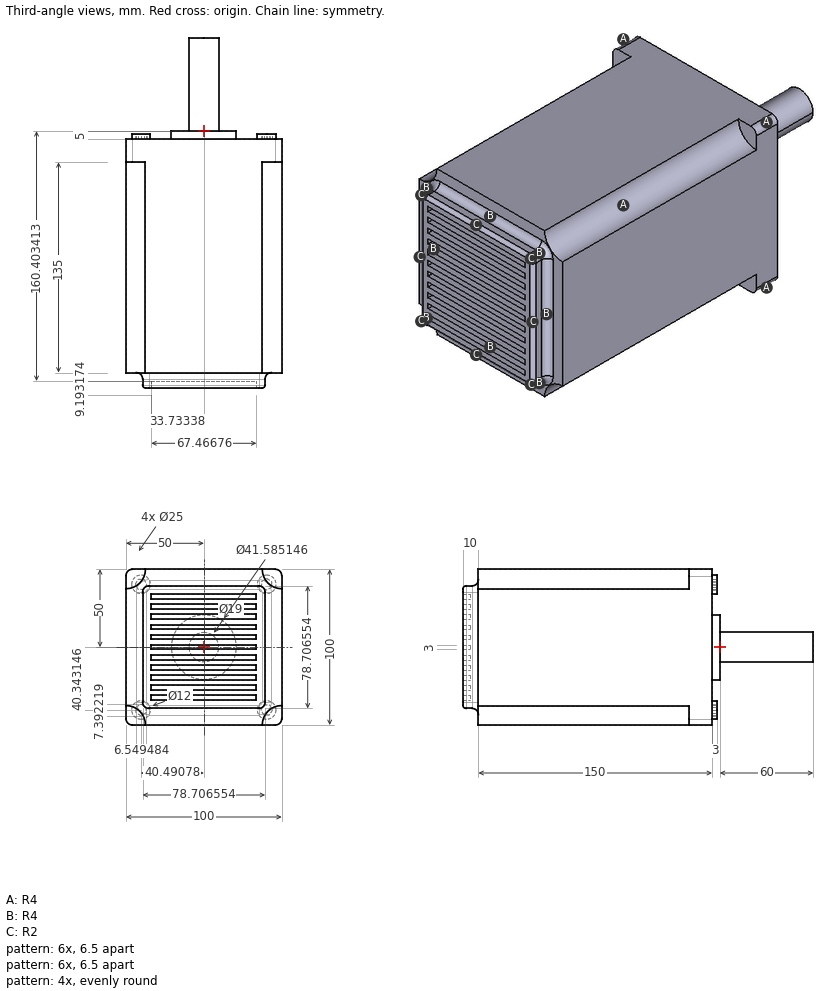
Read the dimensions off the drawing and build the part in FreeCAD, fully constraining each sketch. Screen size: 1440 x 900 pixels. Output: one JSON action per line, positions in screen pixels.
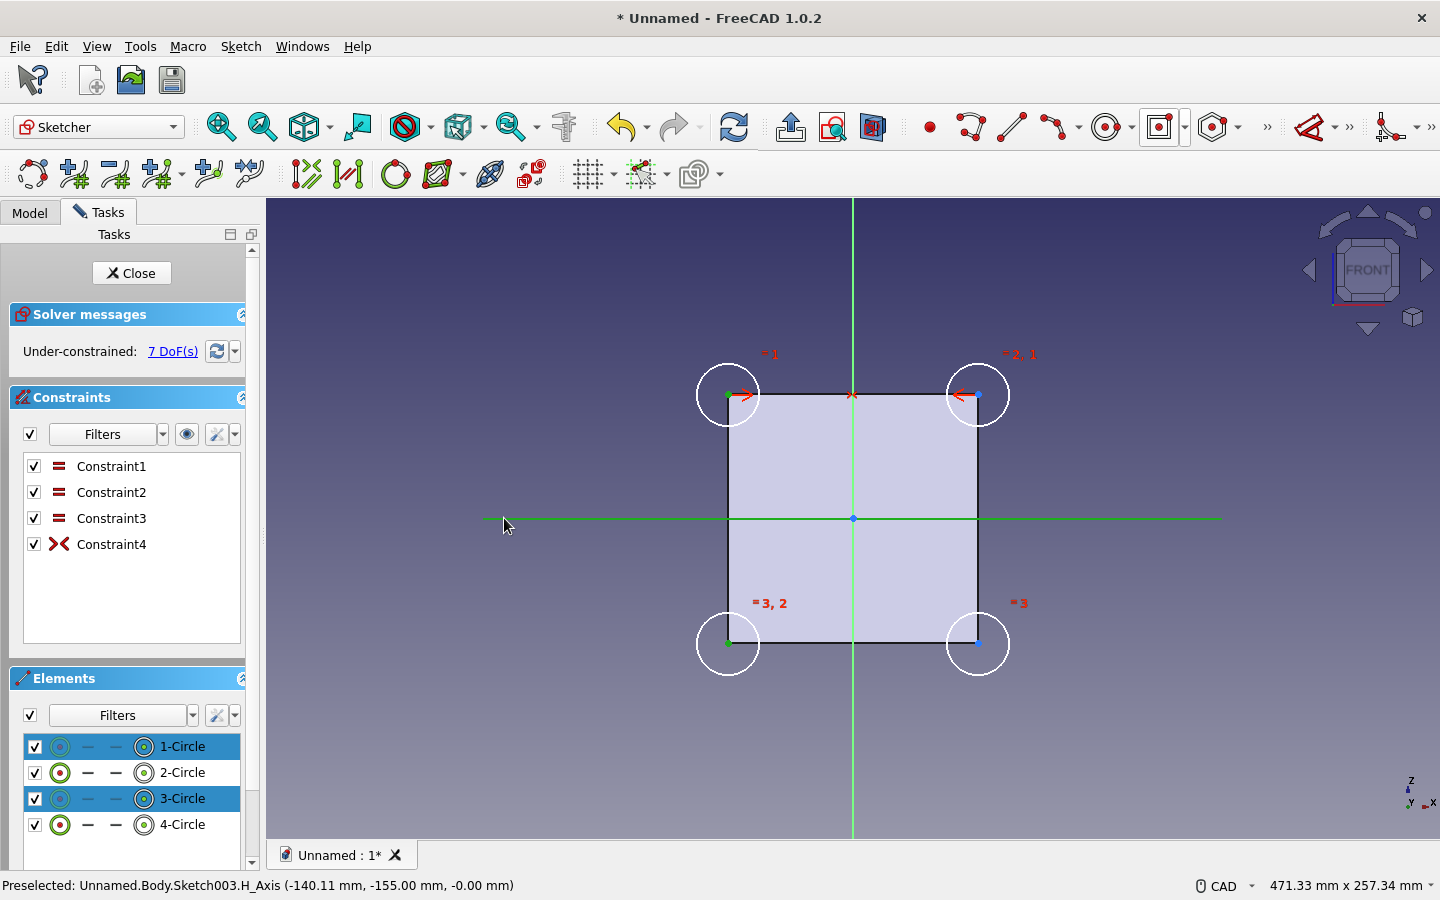
{"action": "key", "text": "s"}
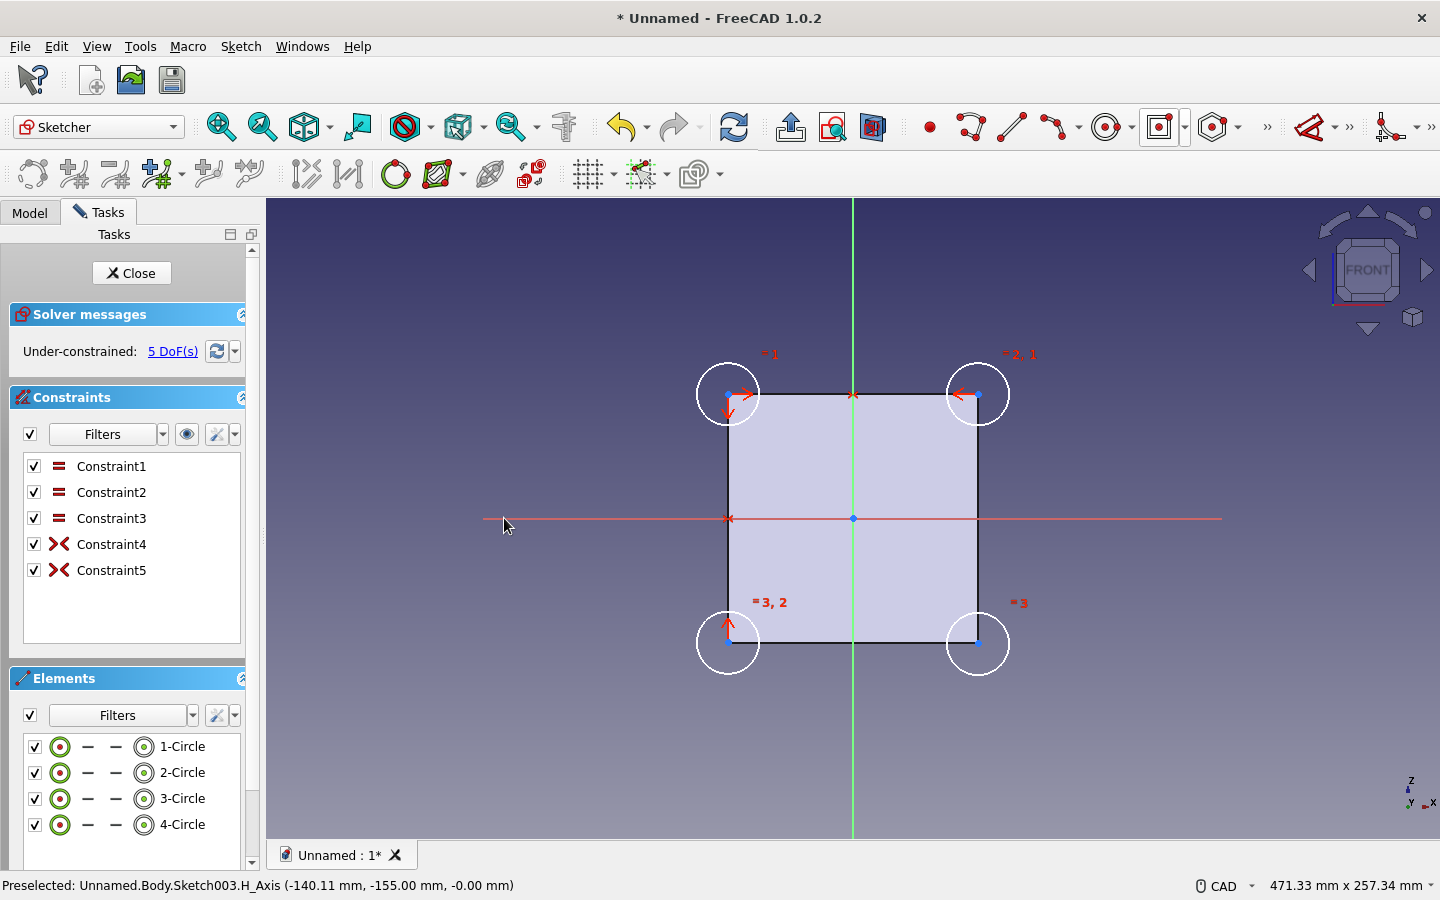
{"action": "left_click", "coordinate": [978, 394]}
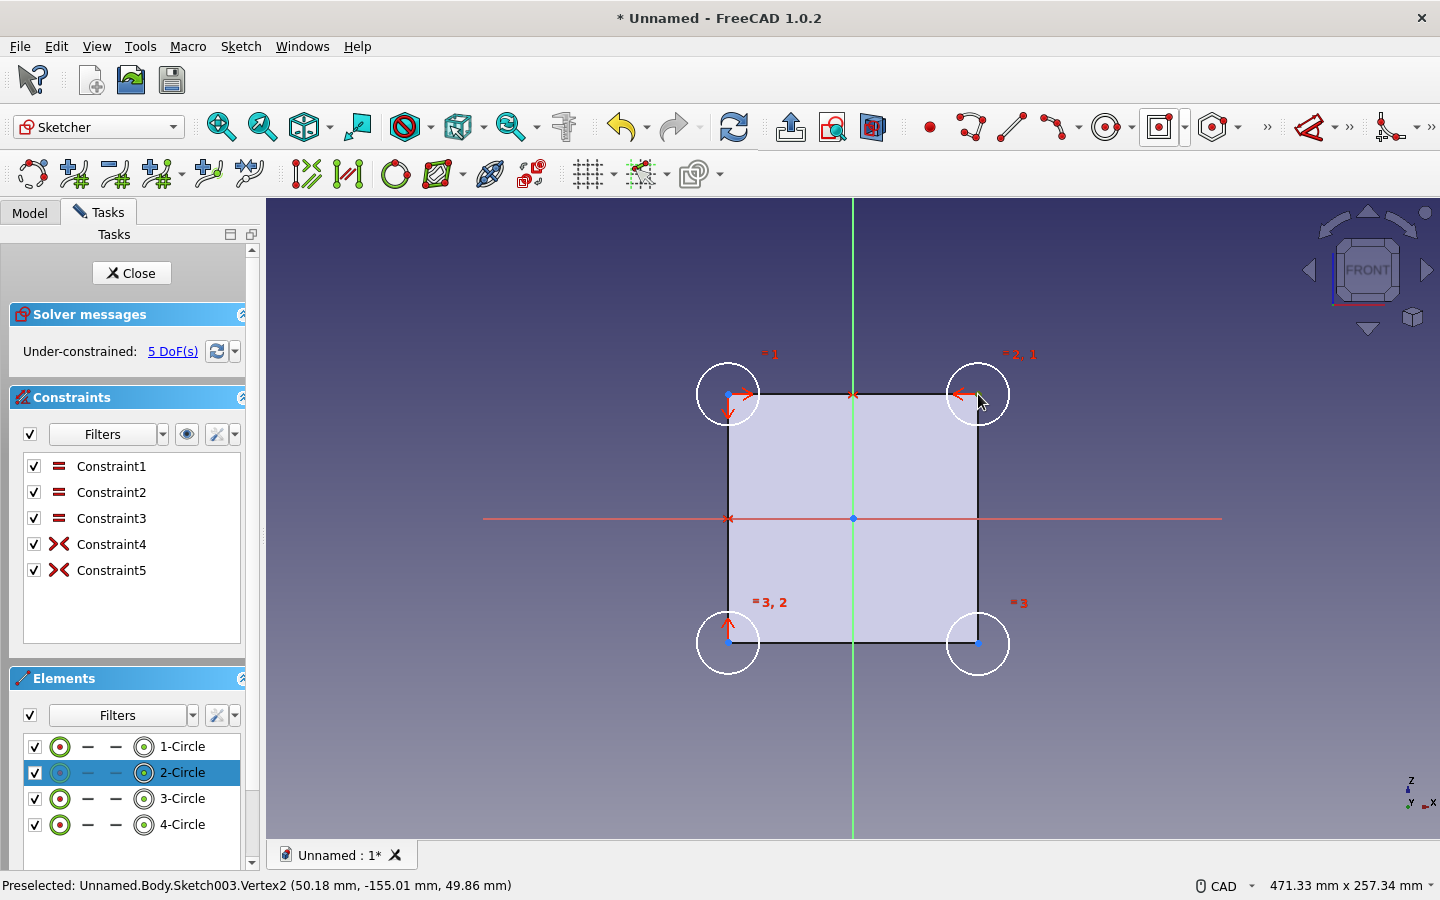
{"action": "left_click", "coordinate": [978, 644]}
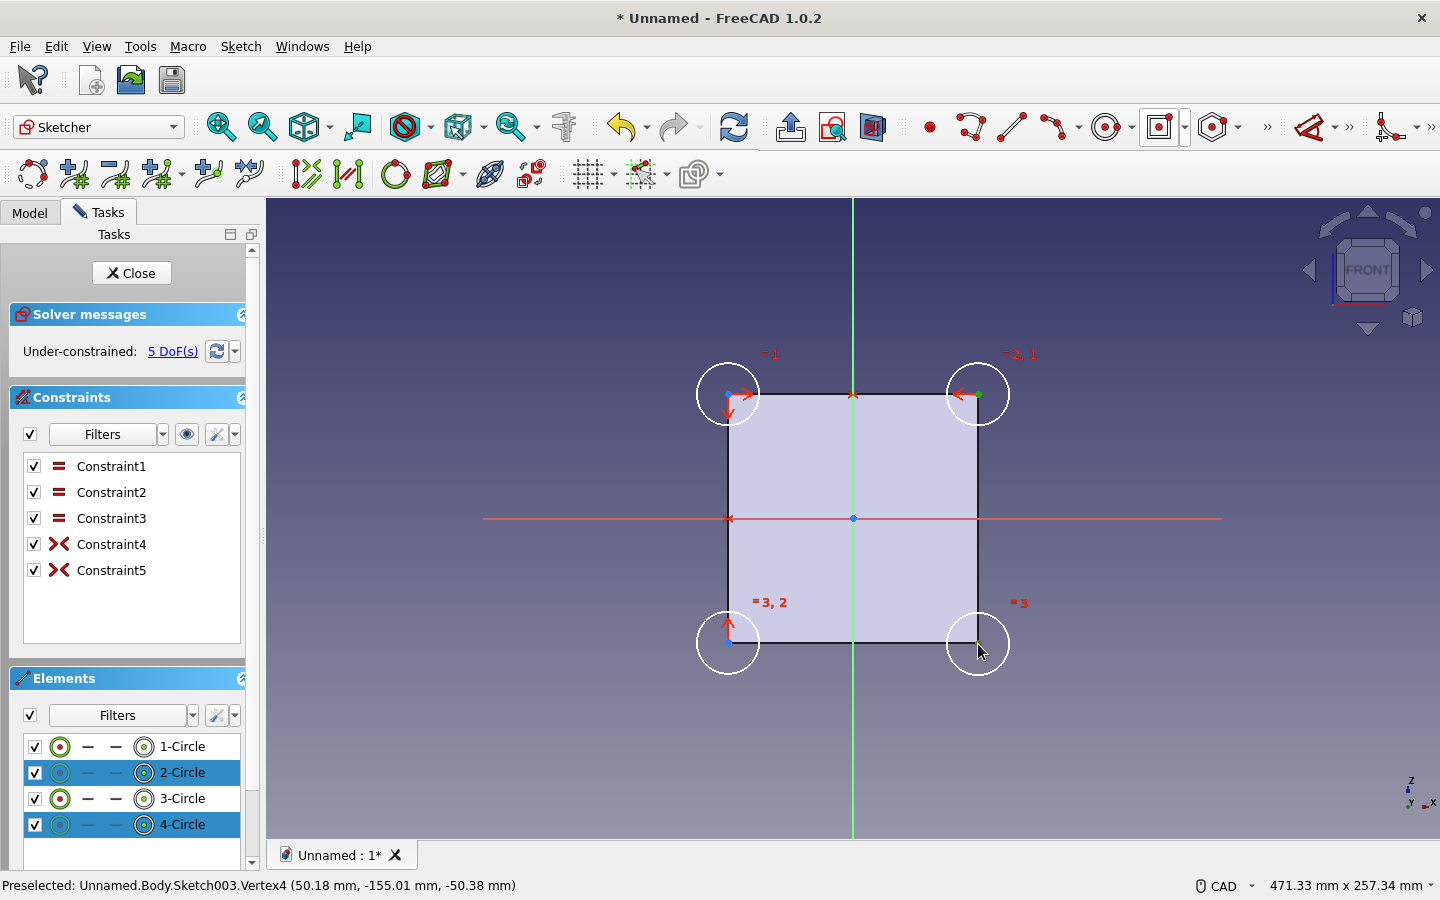
{"action": "left_click", "coordinate": [504, 518]}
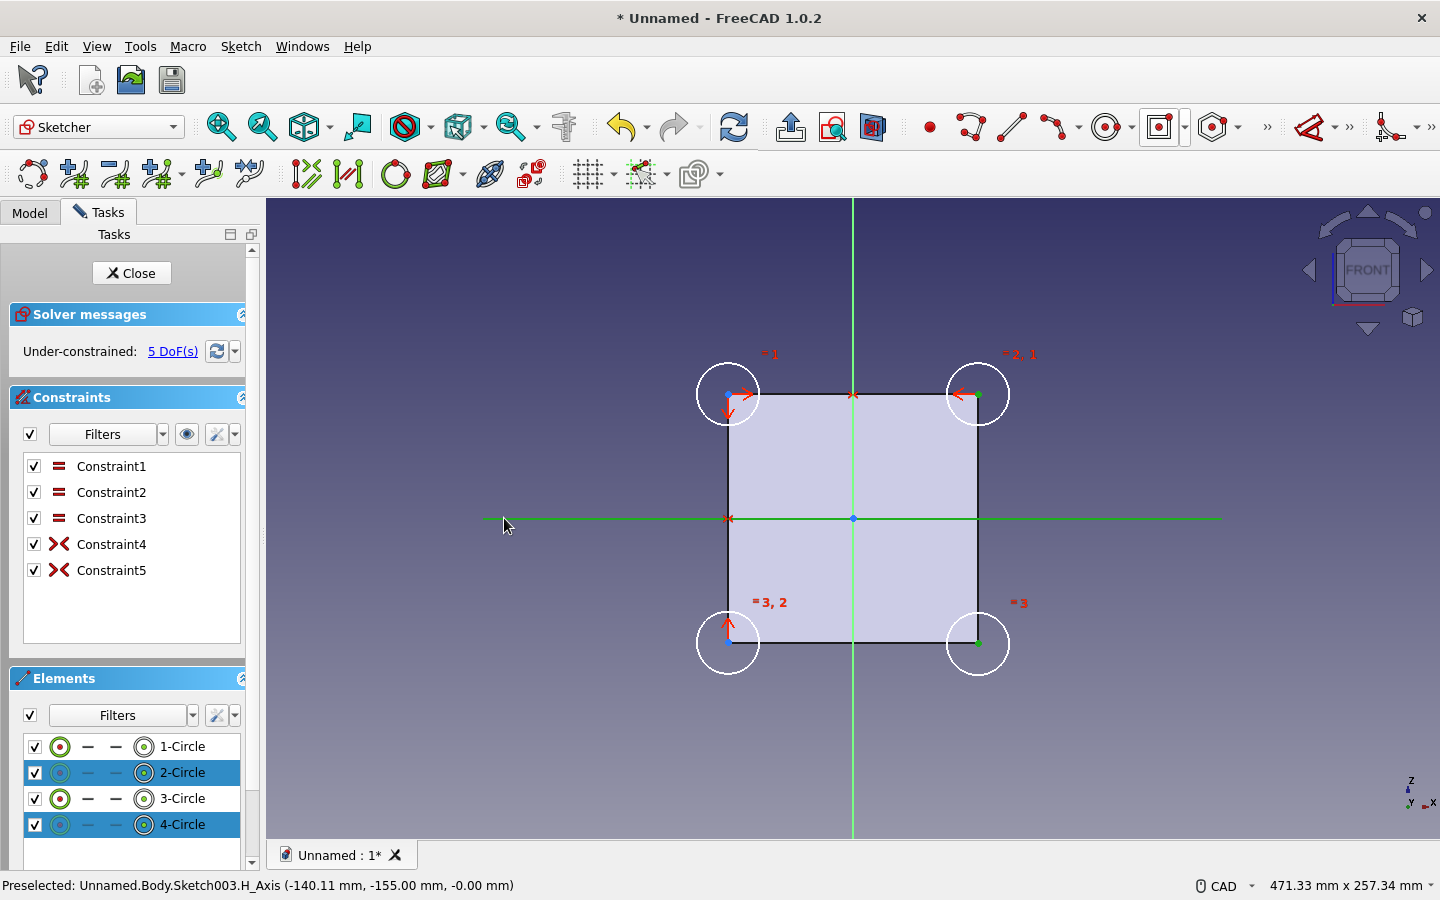
{"action": "key", "text": "s"}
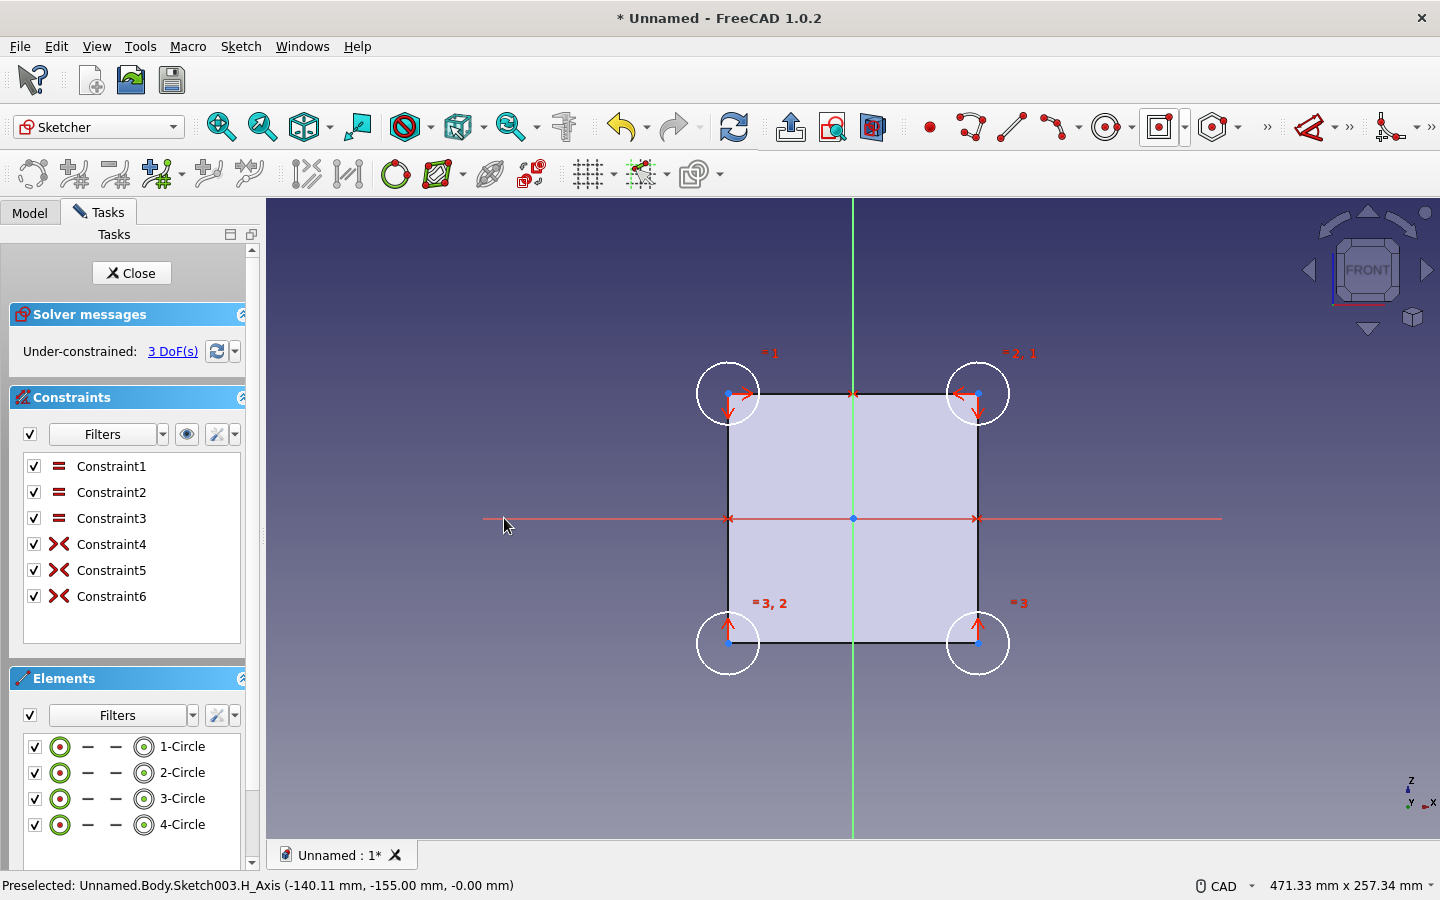
{"action": "left_click", "coordinate": [1308, 128]}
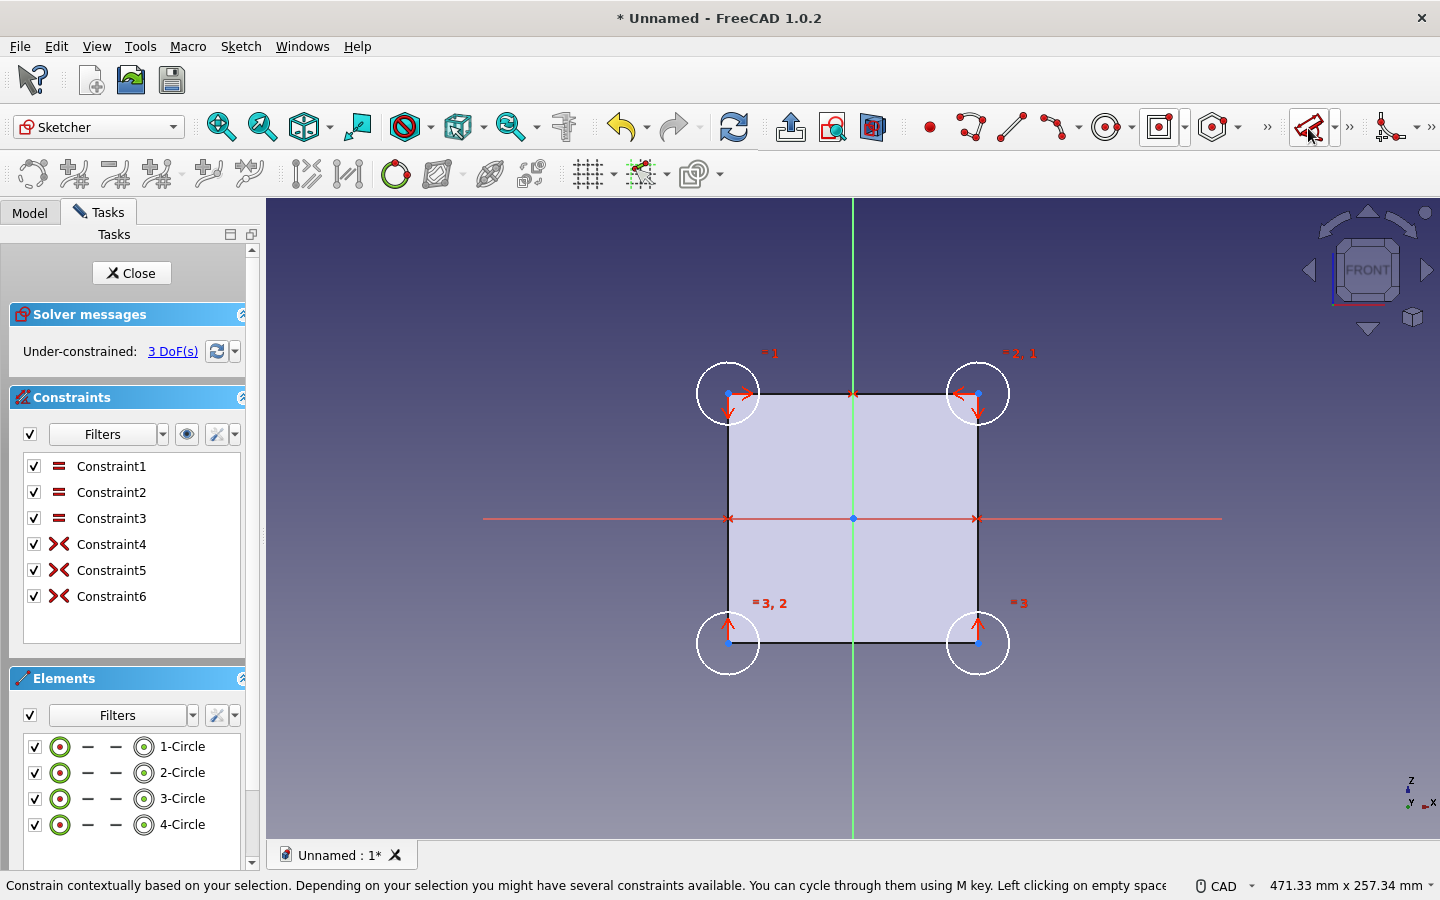
{"action": "left_click", "coordinate": [750, 371]}
{"action": "left_click", "coordinate": [772, 348]}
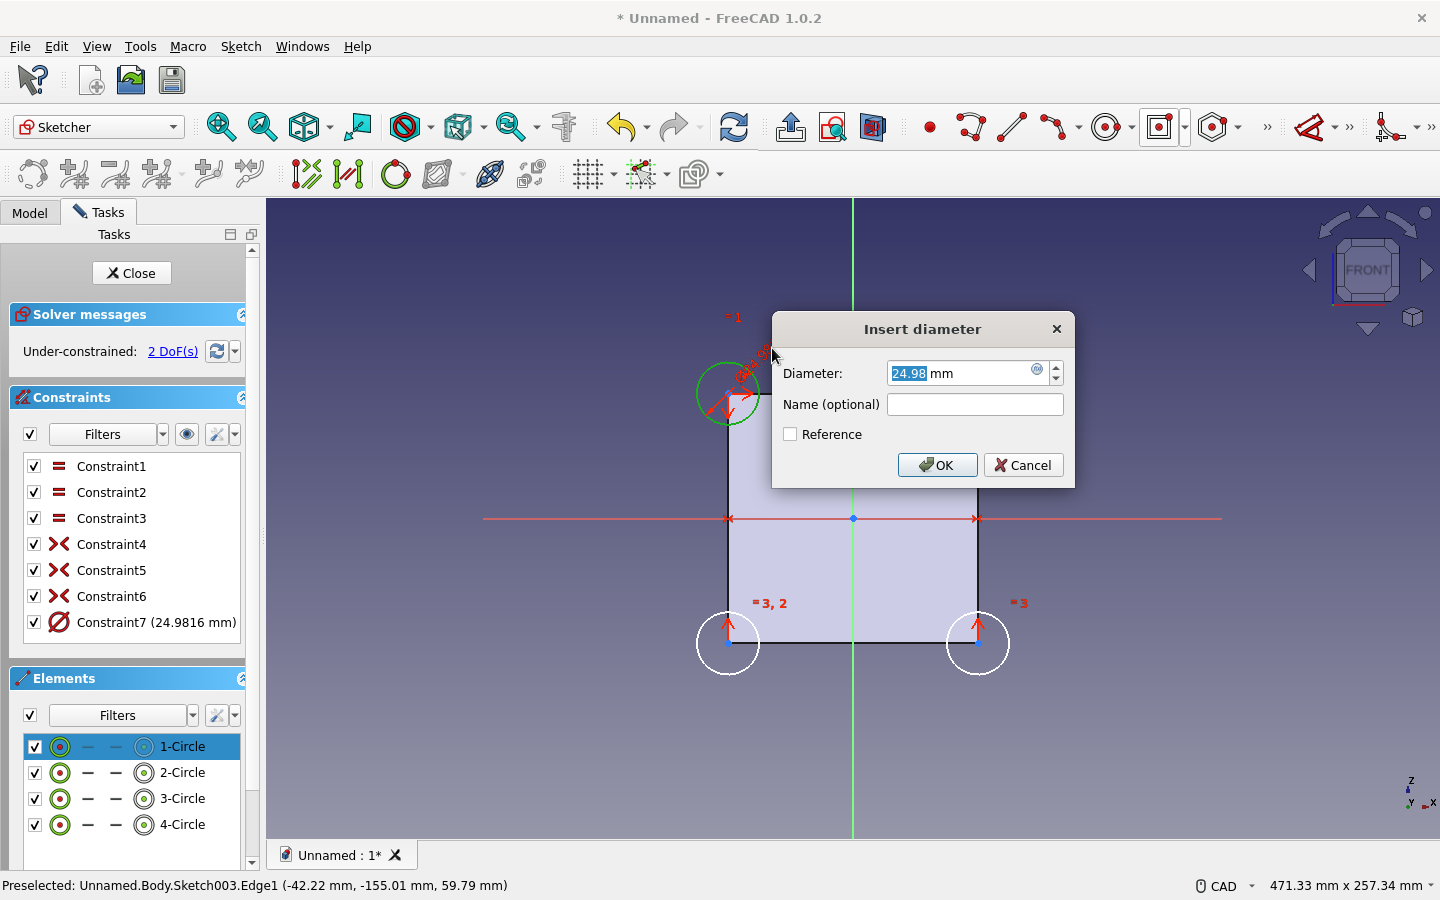
{"action": "type", "text": "25"}
{"action": "key", "text": "Return"}